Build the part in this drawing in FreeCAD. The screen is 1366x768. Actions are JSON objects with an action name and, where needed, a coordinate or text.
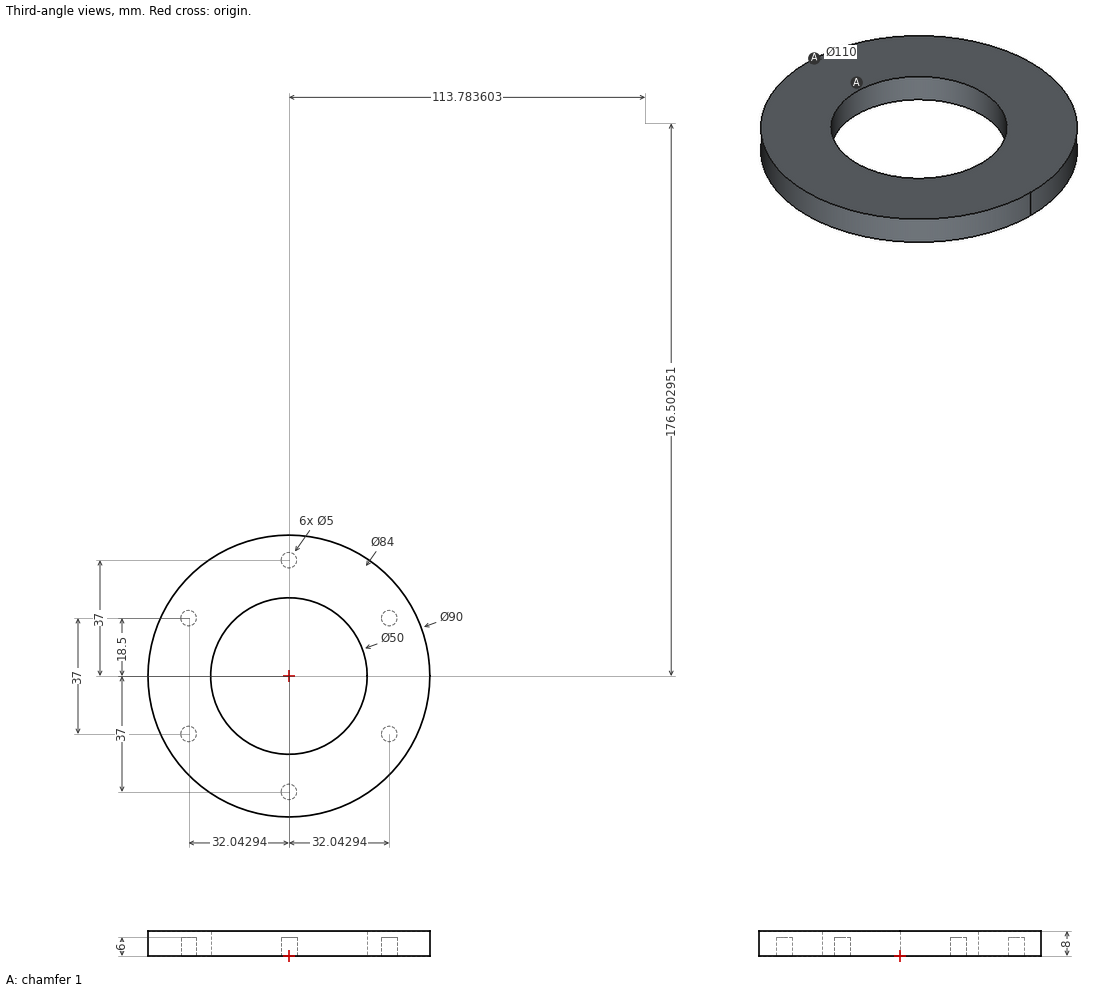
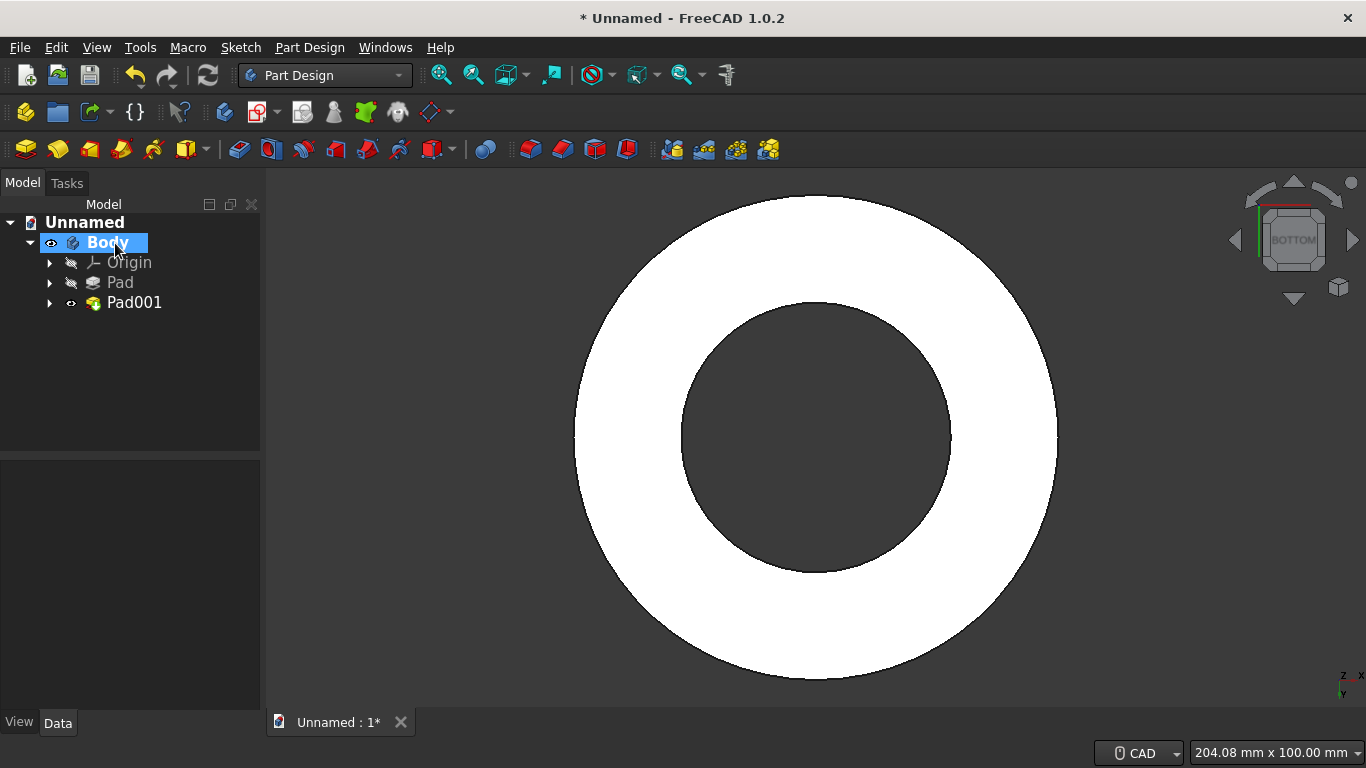
{"action": "left_click", "coordinate": [955, 575]}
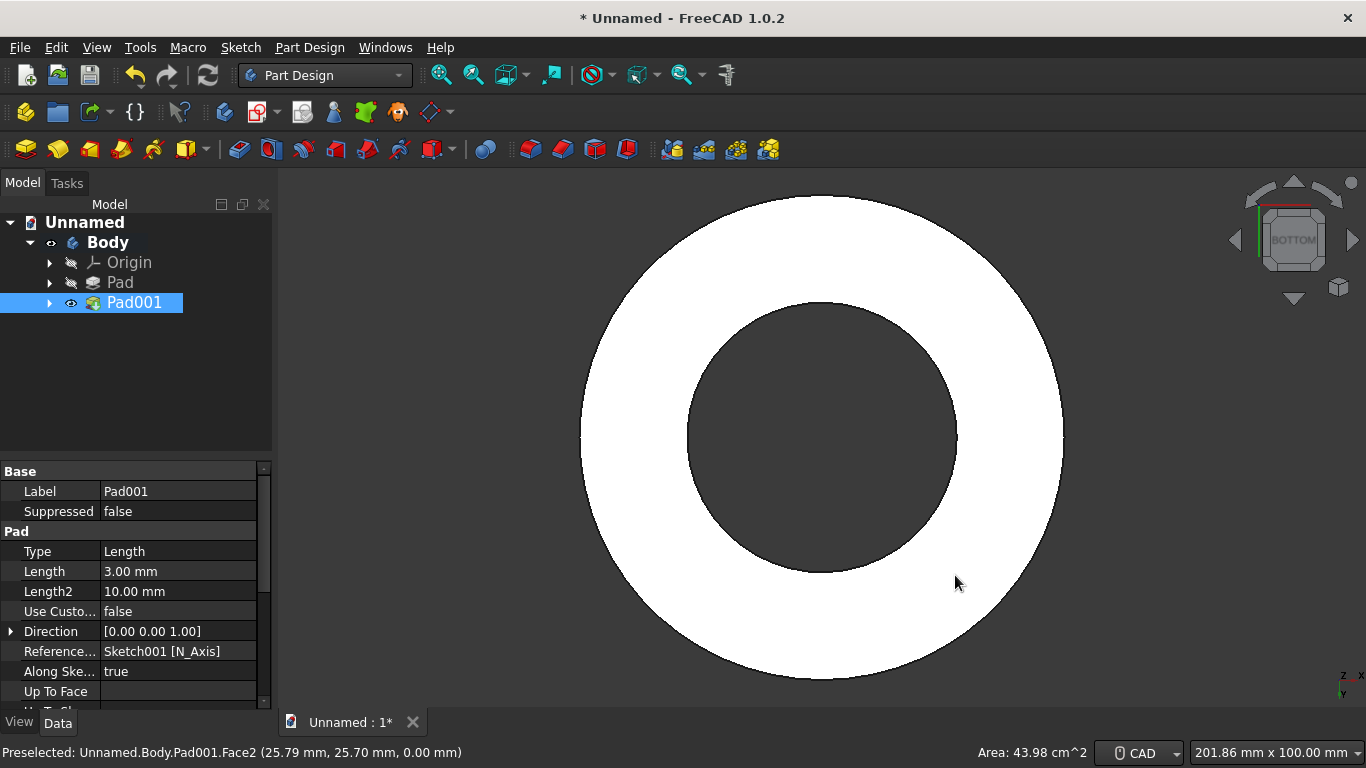
{"action": "left_click", "coordinate": [258, 112]}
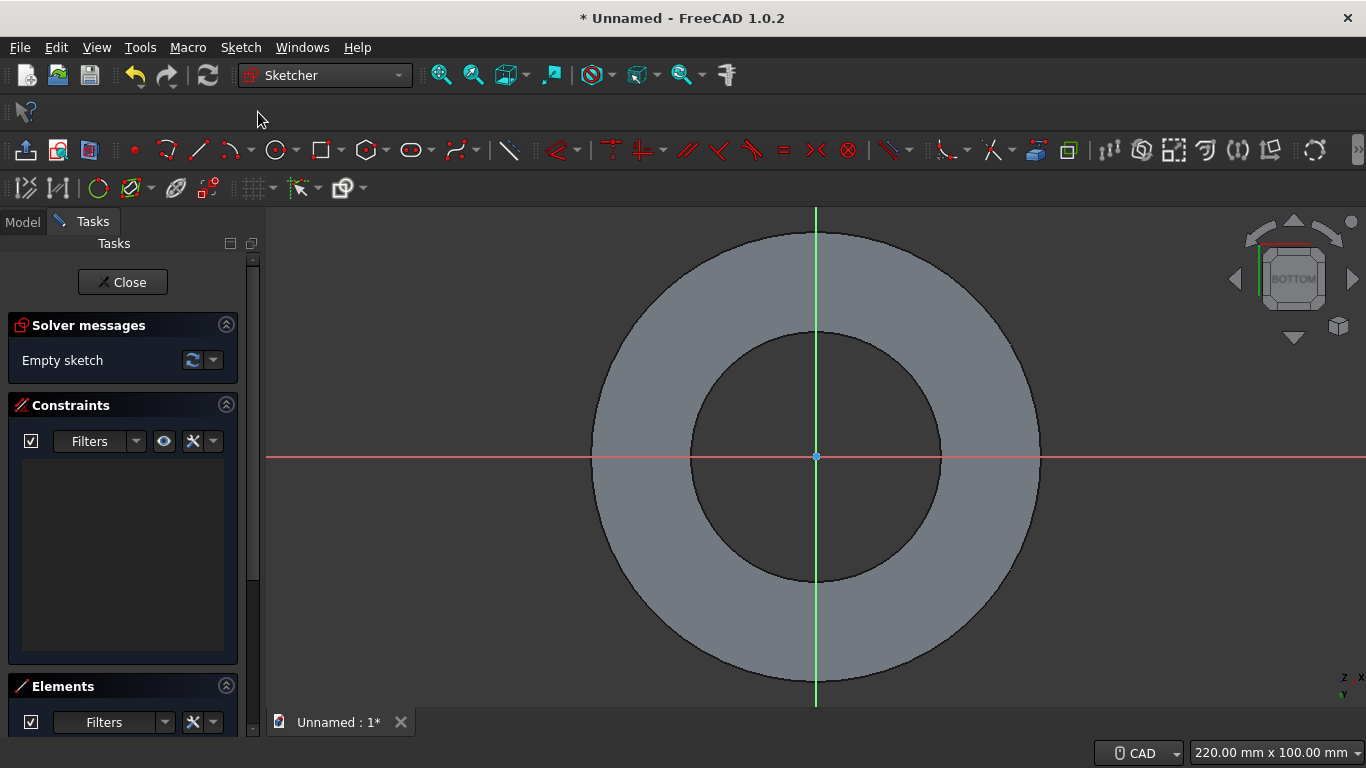
{"action": "scroll", "coordinate": [438, 457], "scroll_direction": "down", "scroll_amount": 1}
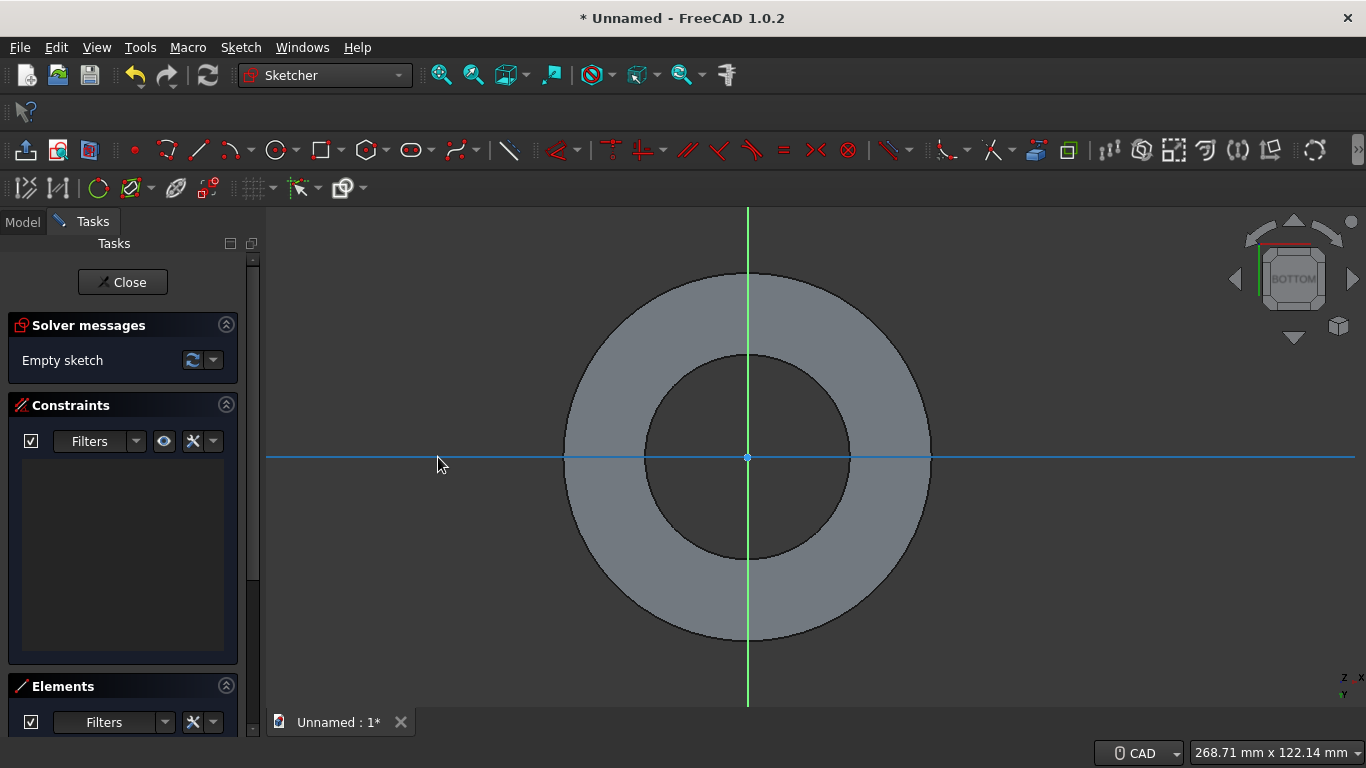
{"action": "key", "text": "g c"}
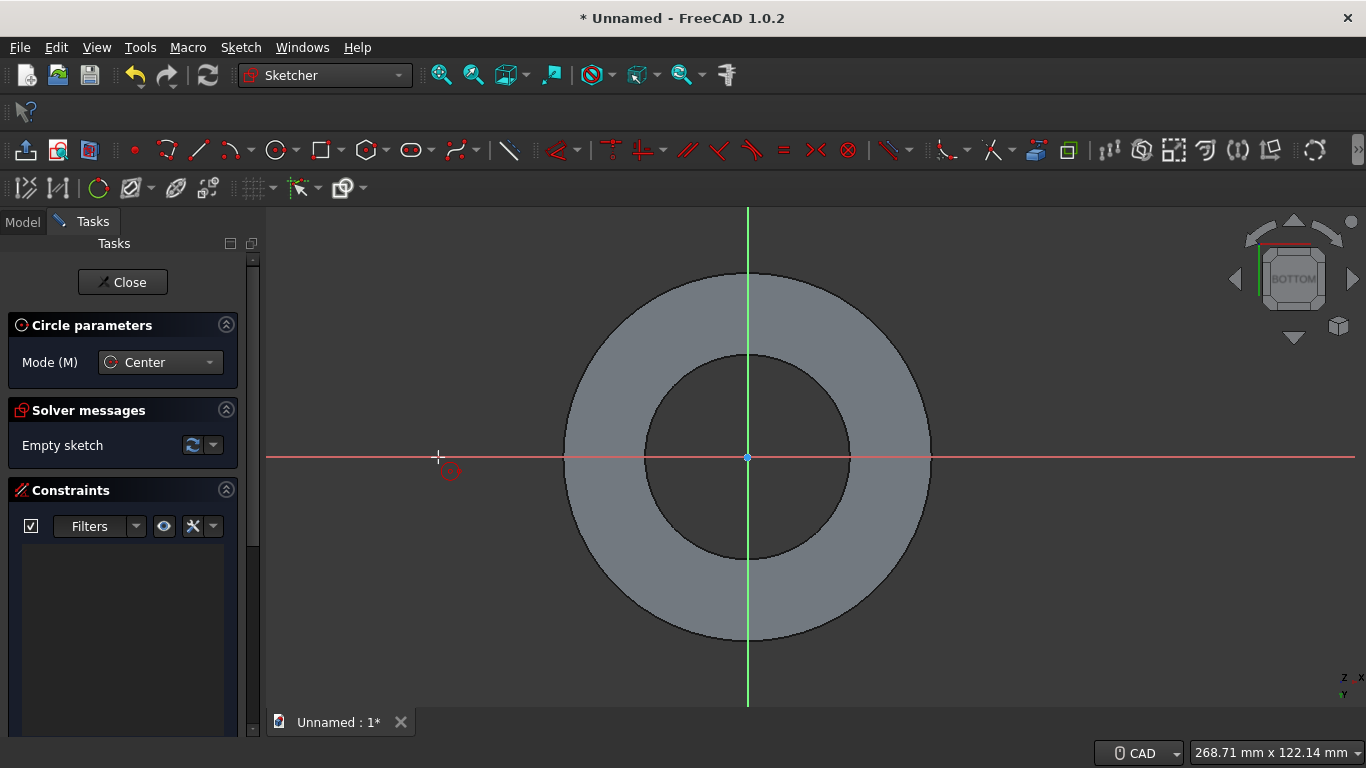
{"action": "scroll", "coordinate": [748, 609], "scroll_direction": "up", "scroll_amount": 4}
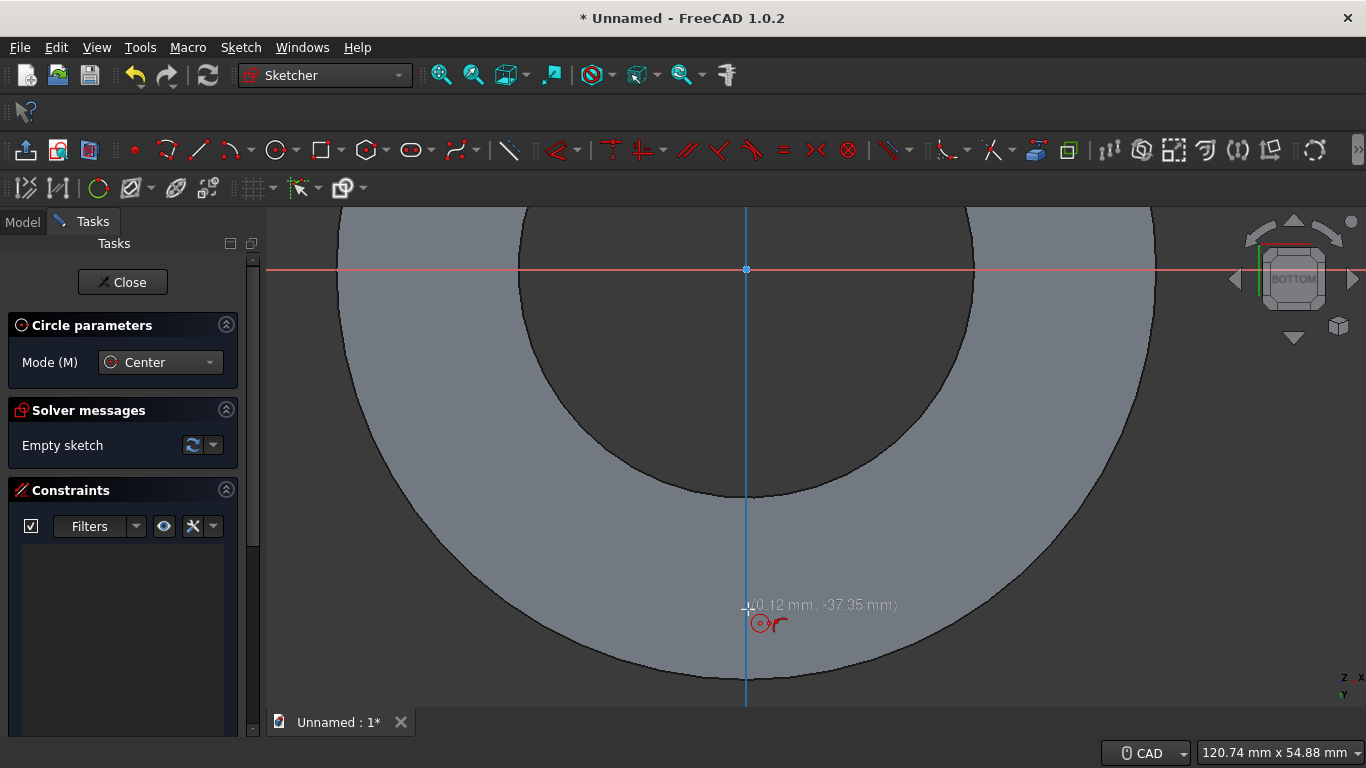
{"action": "left_click", "coordinate": [746, 607]}
{"action": "mouse_move", "coordinate": [762, 591]}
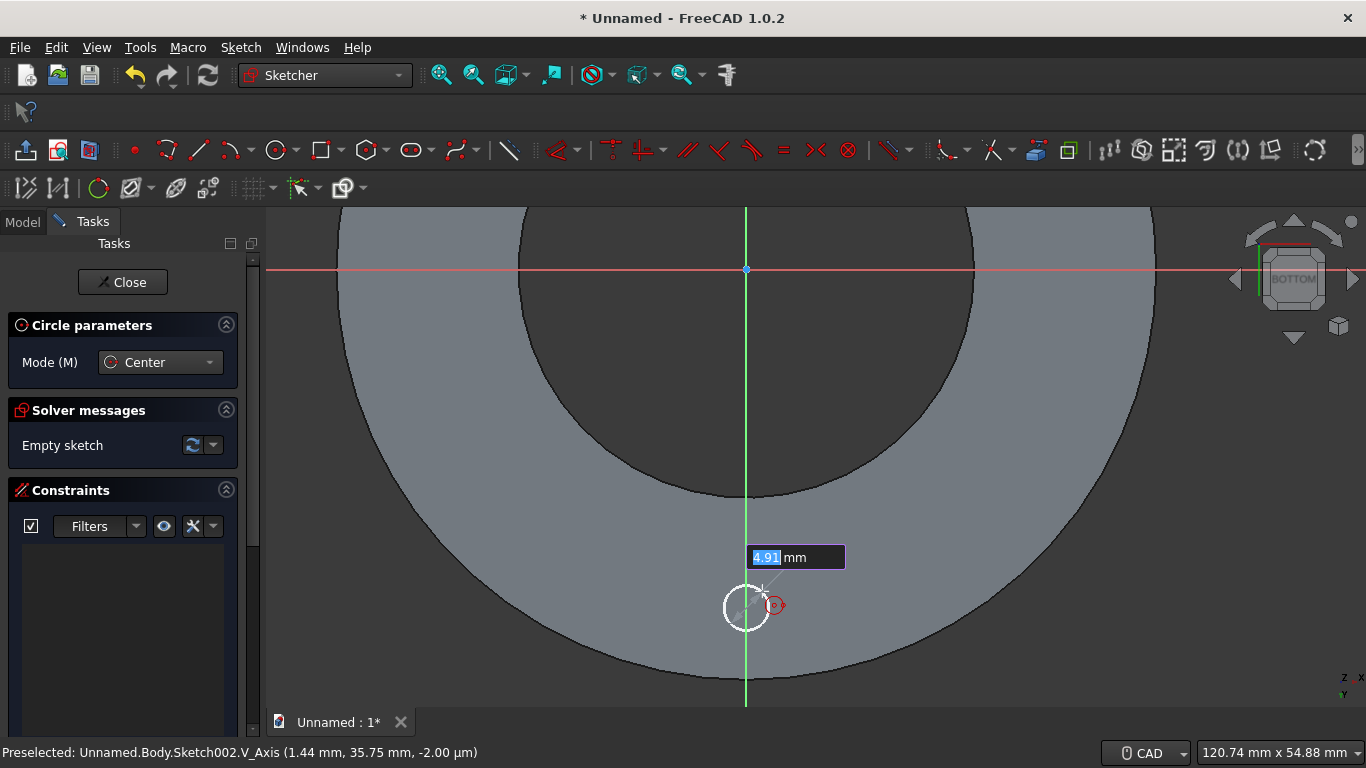
{"action": "type", "text": "5"}
{"action": "key", "text": "Return"}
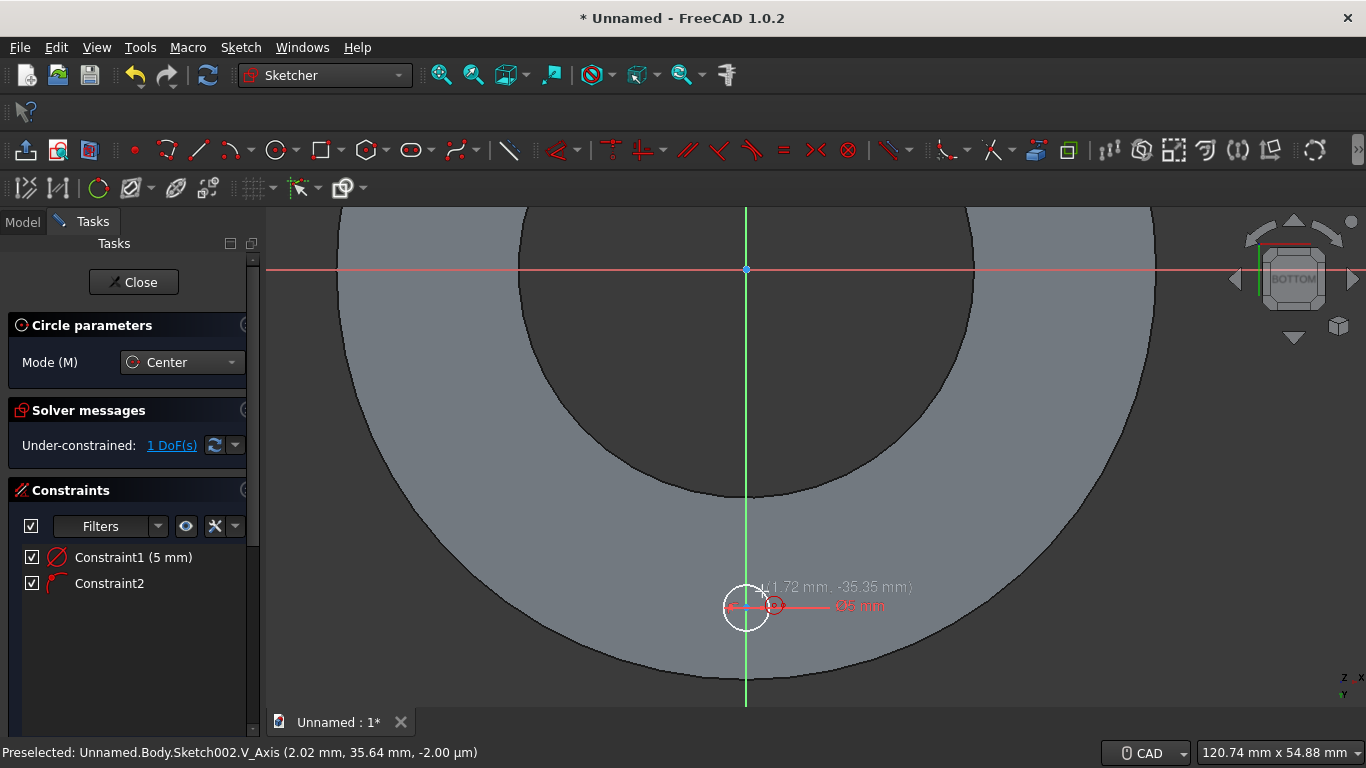
{"action": "left_click", "coordinate": [454, 438]}
{"action": "mouse_move", "coordinate": [471, 422]}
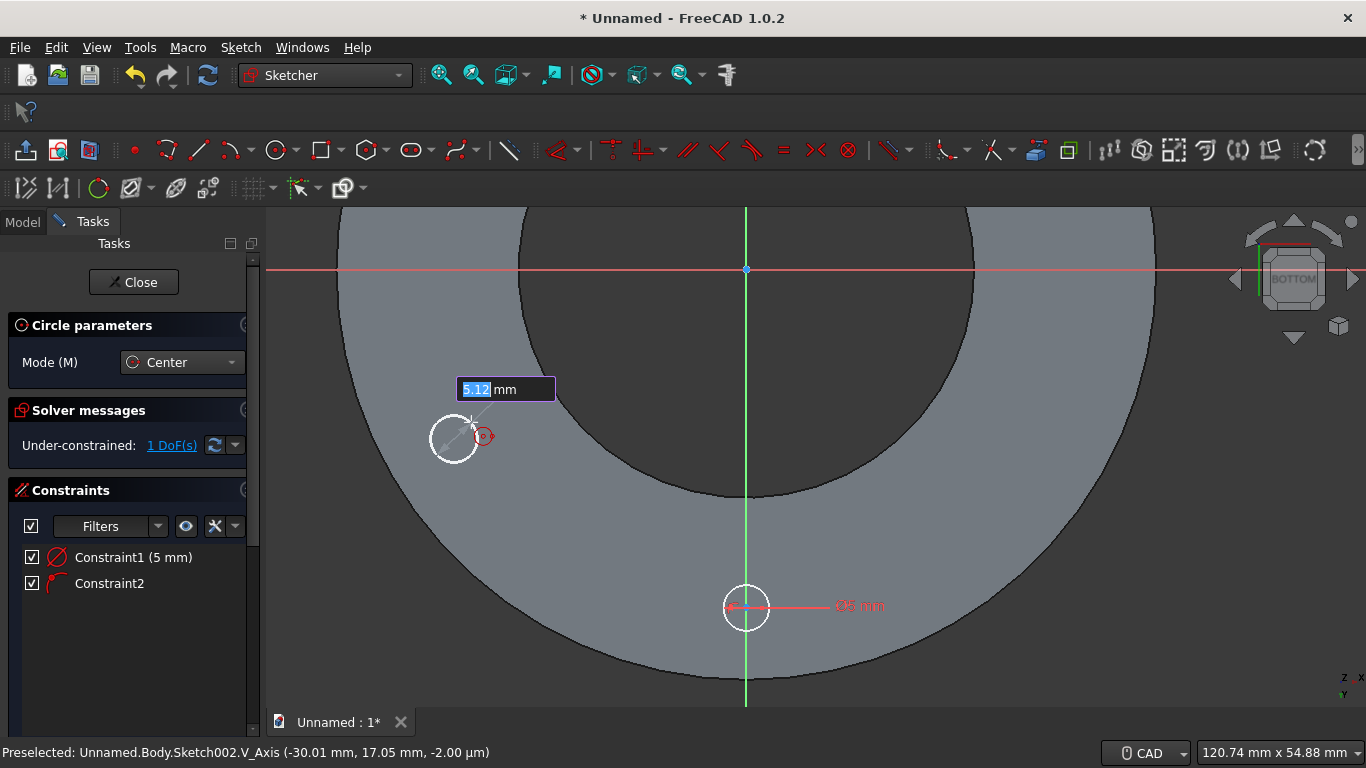
{"action": "type", "text": "5"}
{"action": "key", "text": "Return"}